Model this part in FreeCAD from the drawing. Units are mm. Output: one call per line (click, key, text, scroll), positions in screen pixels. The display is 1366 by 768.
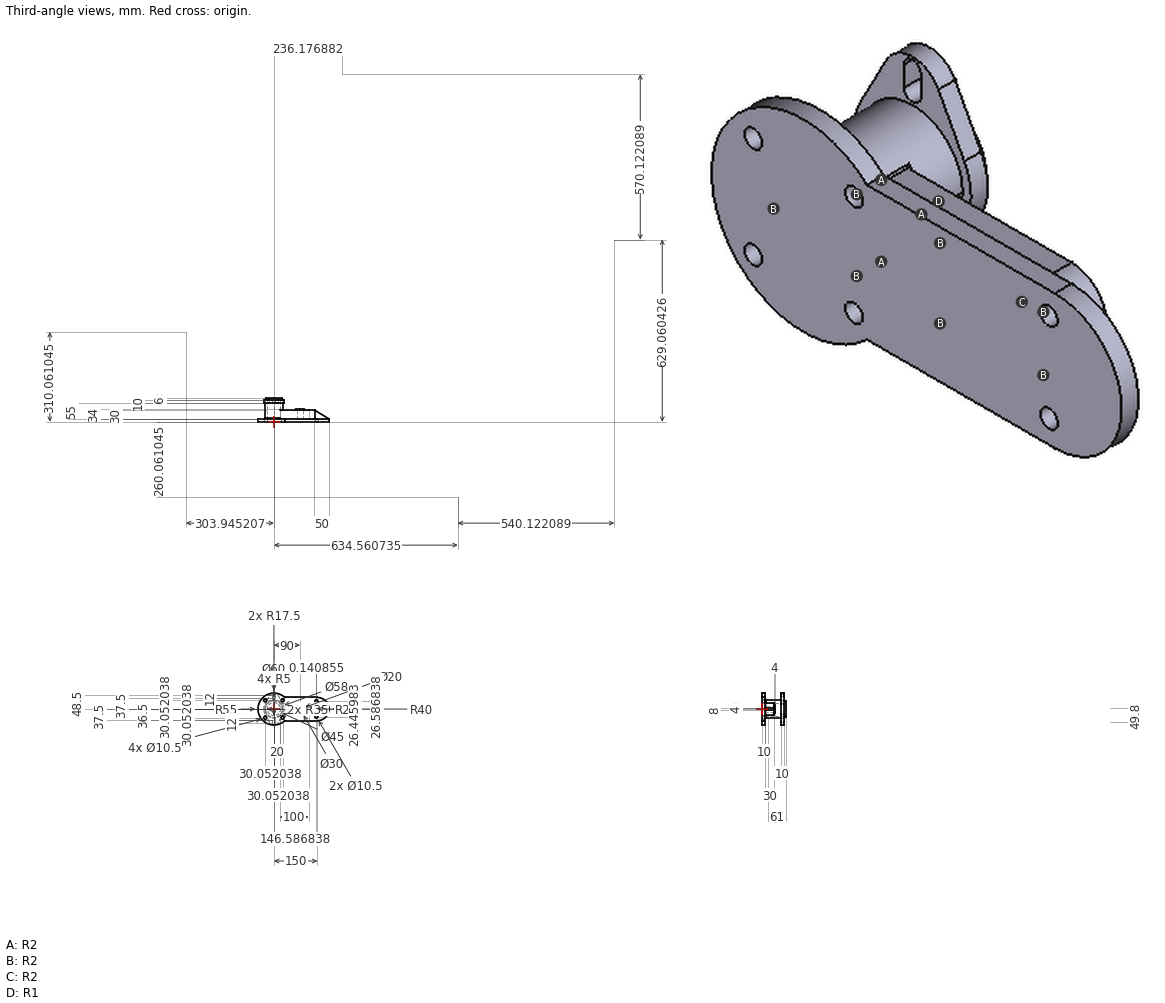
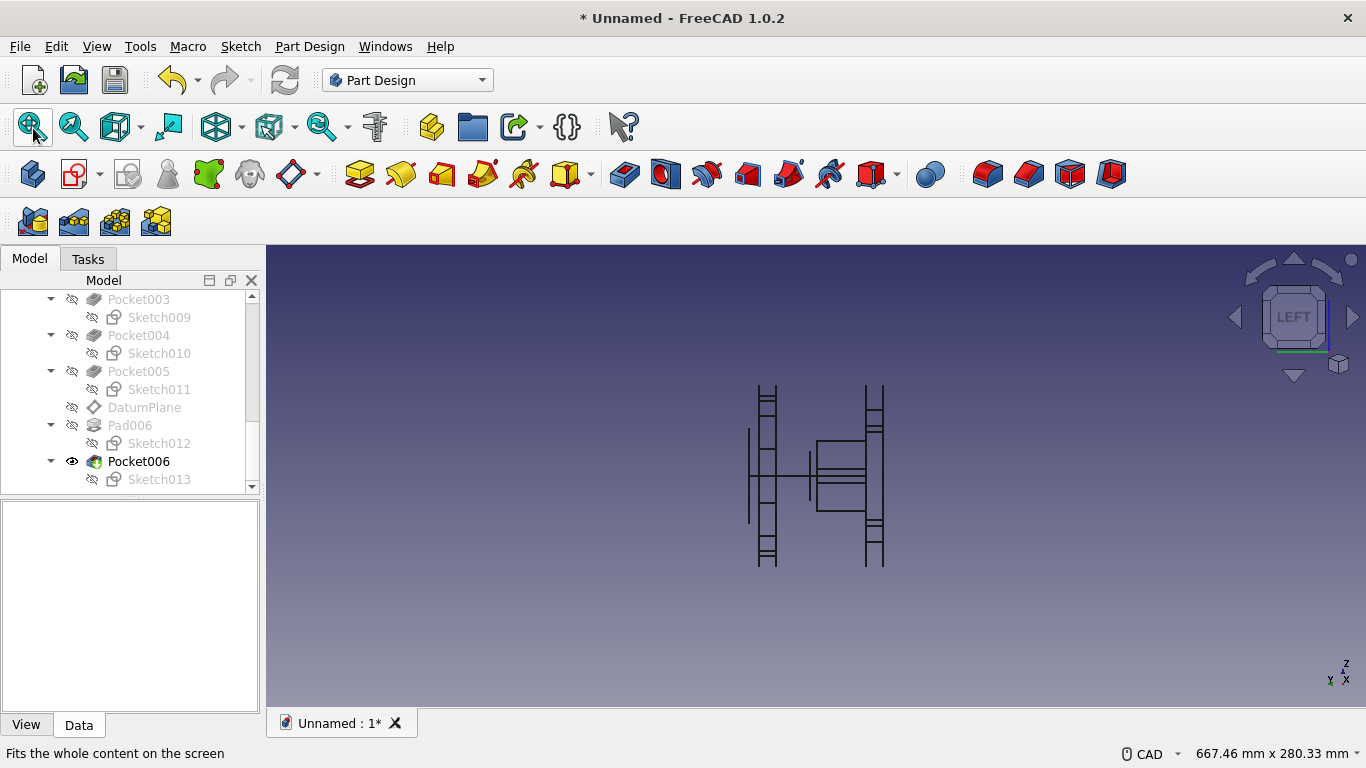
key(0)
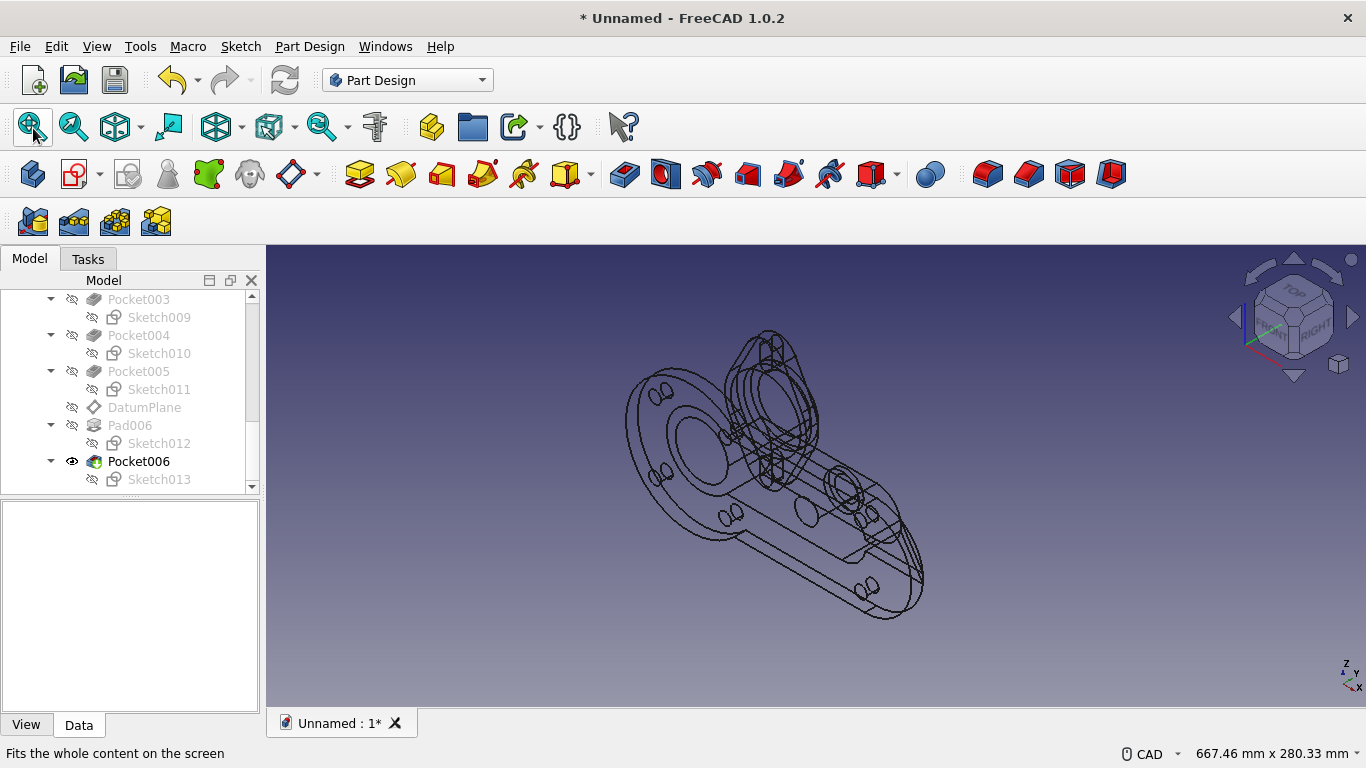
click(757, 418)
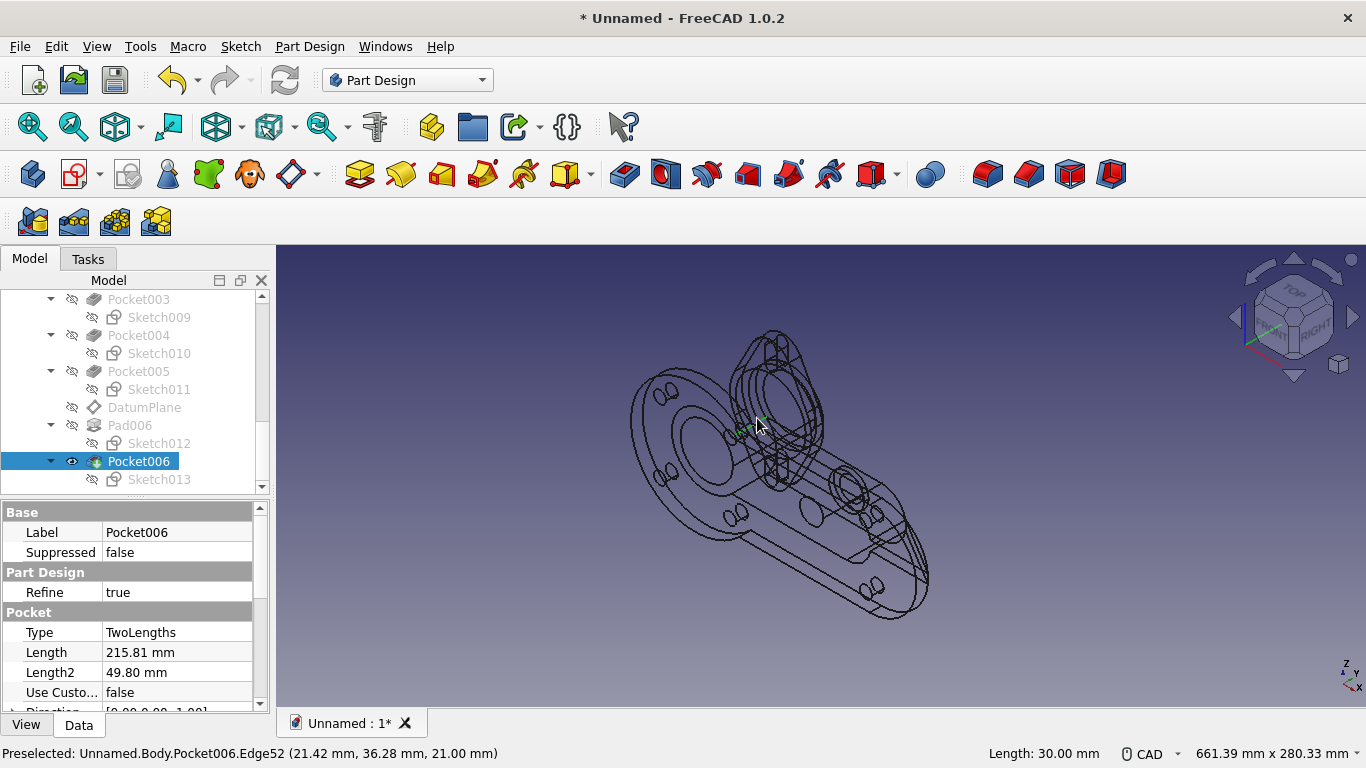
click(749, 483, ctrl)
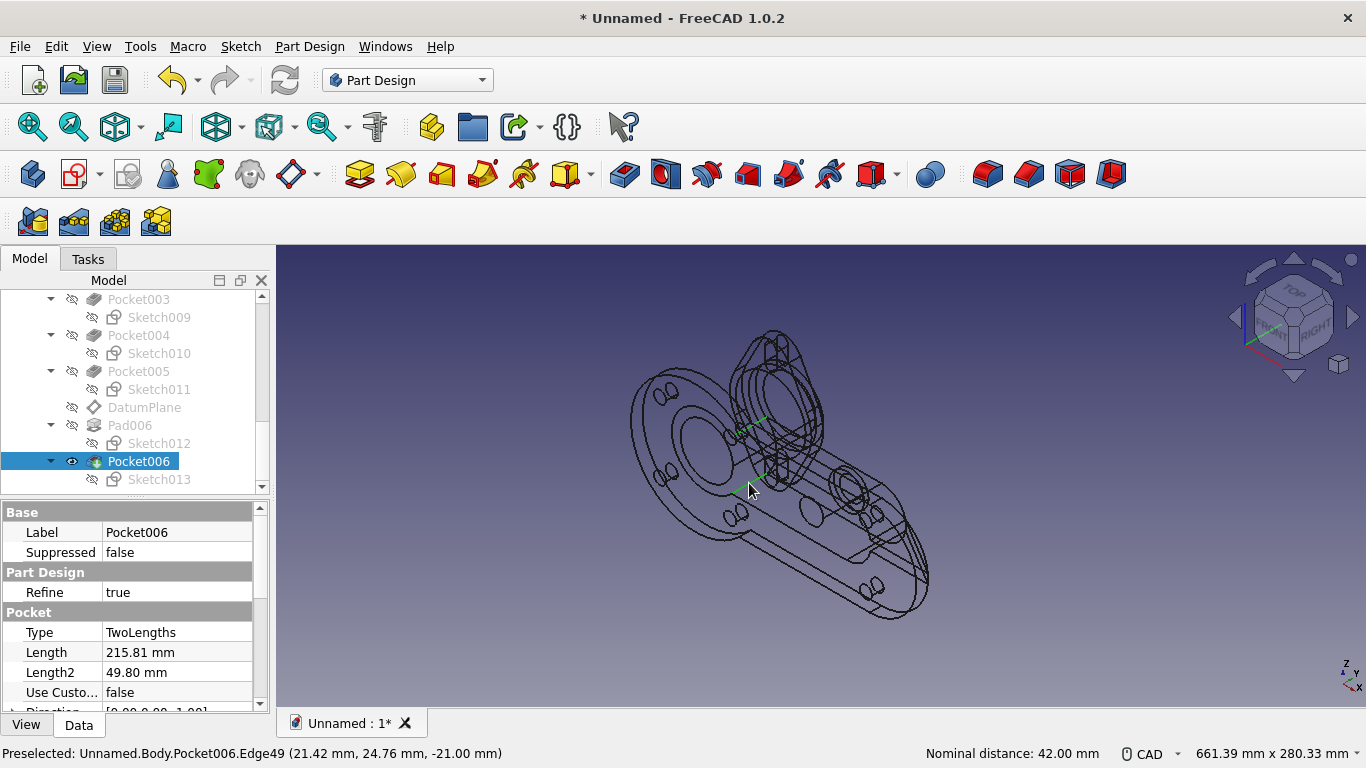
click(772, 468, ctrl)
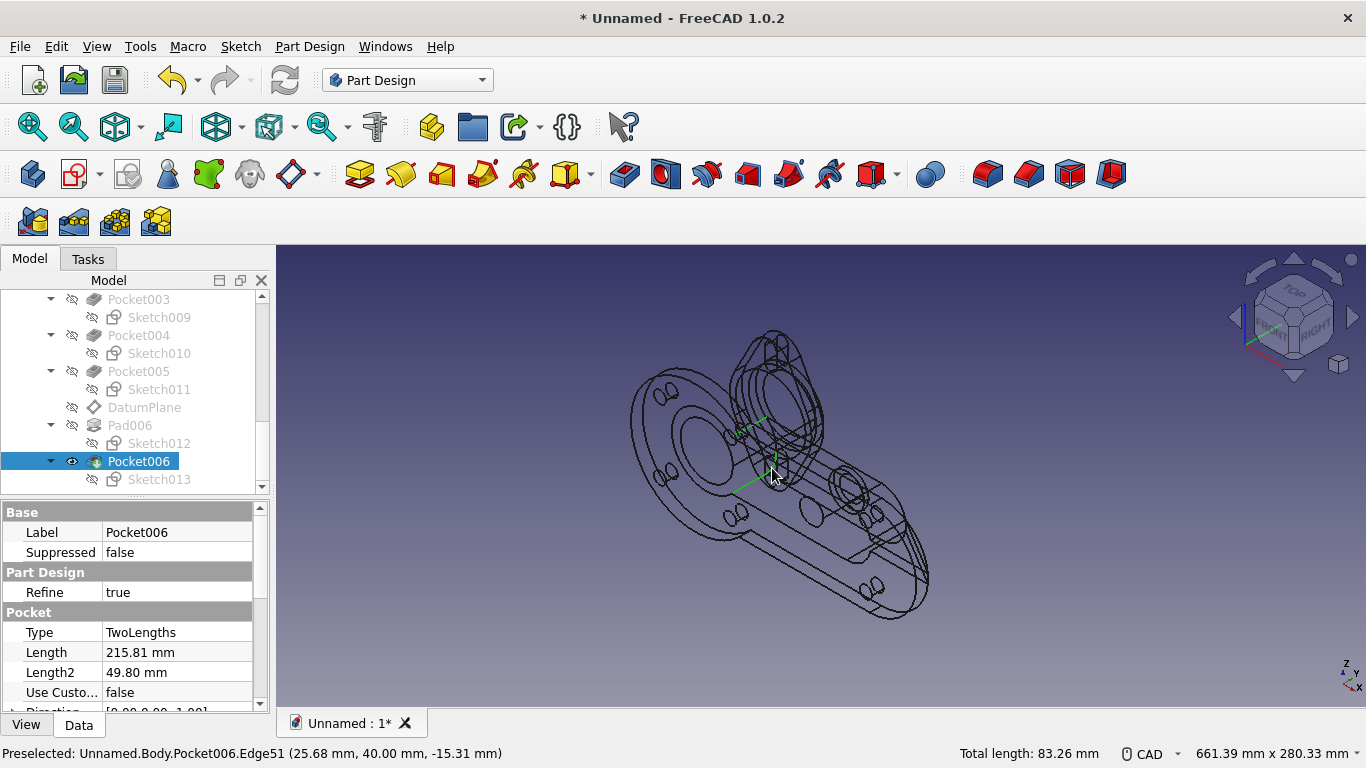
key(v)
key(1)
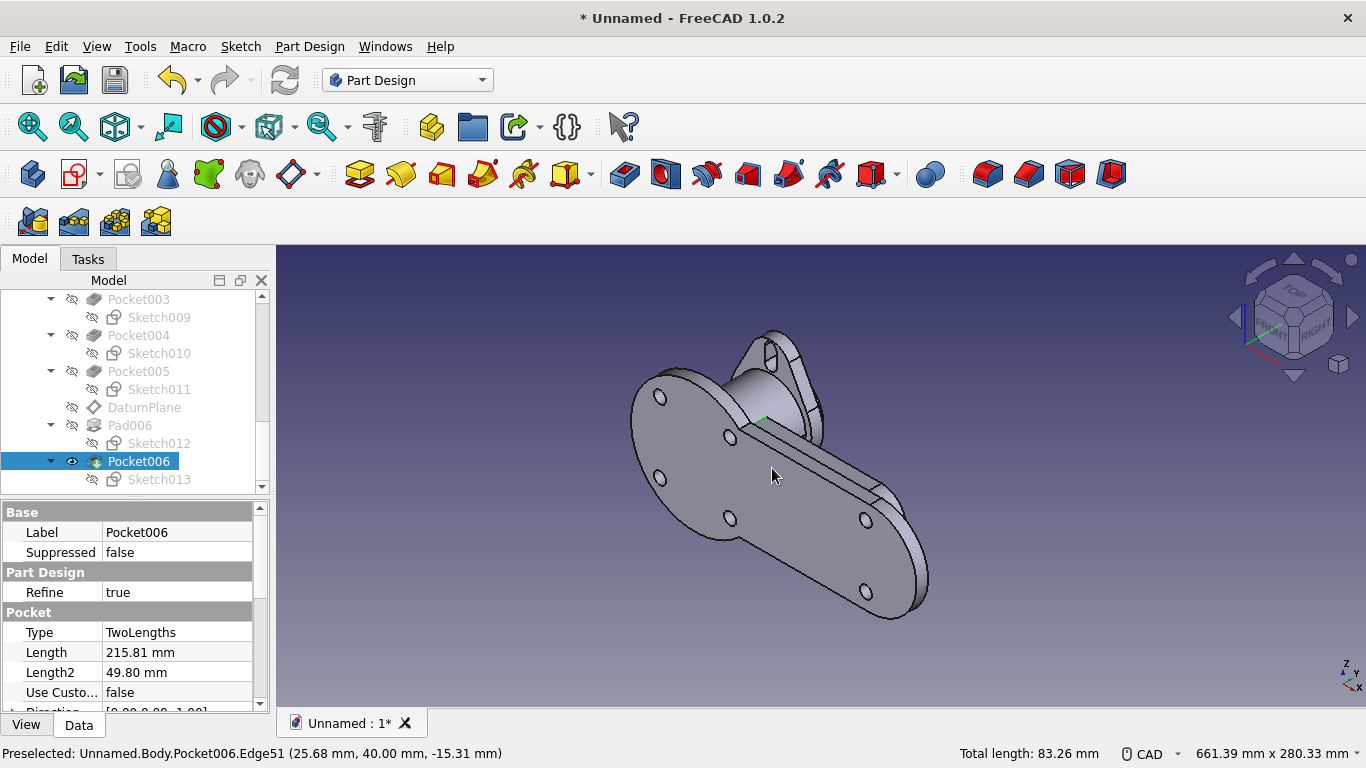
click(988, 174)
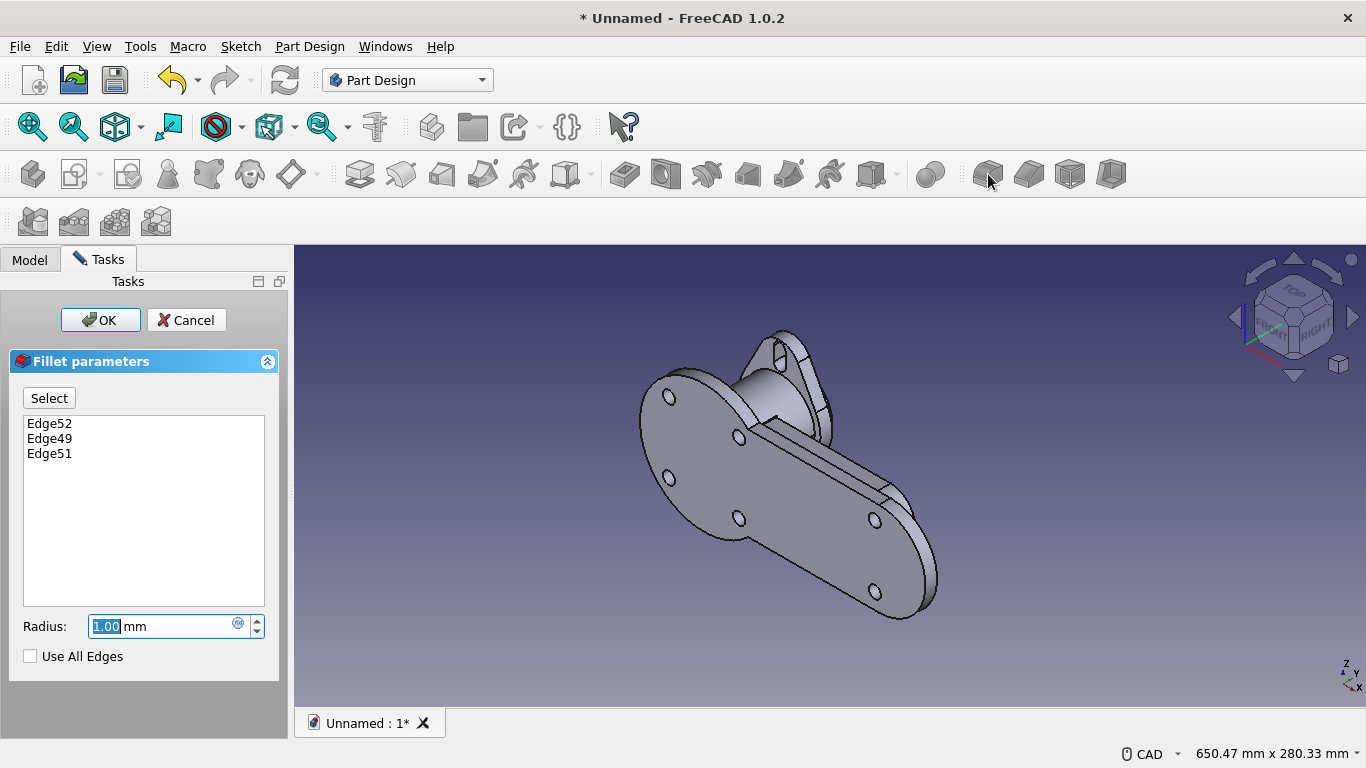
text(2)
key(Tab)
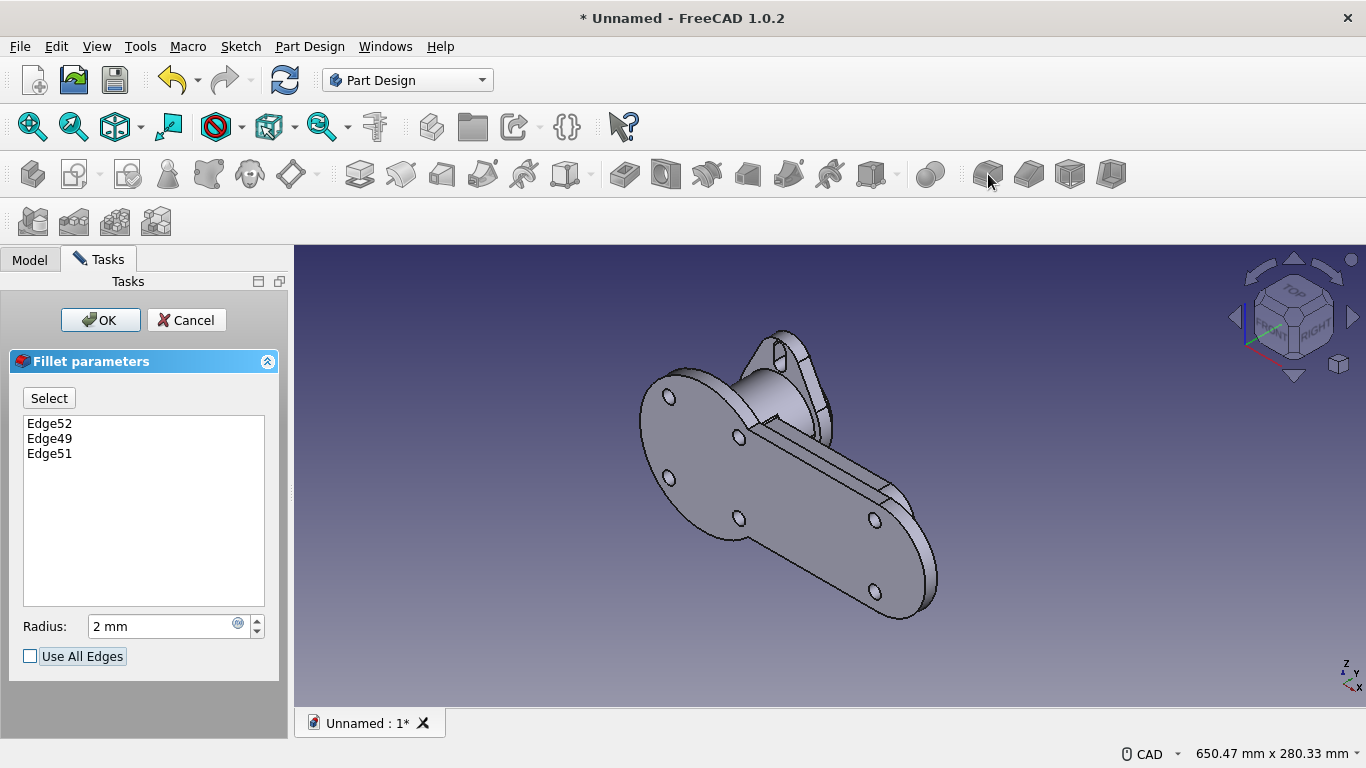
click(101, 320)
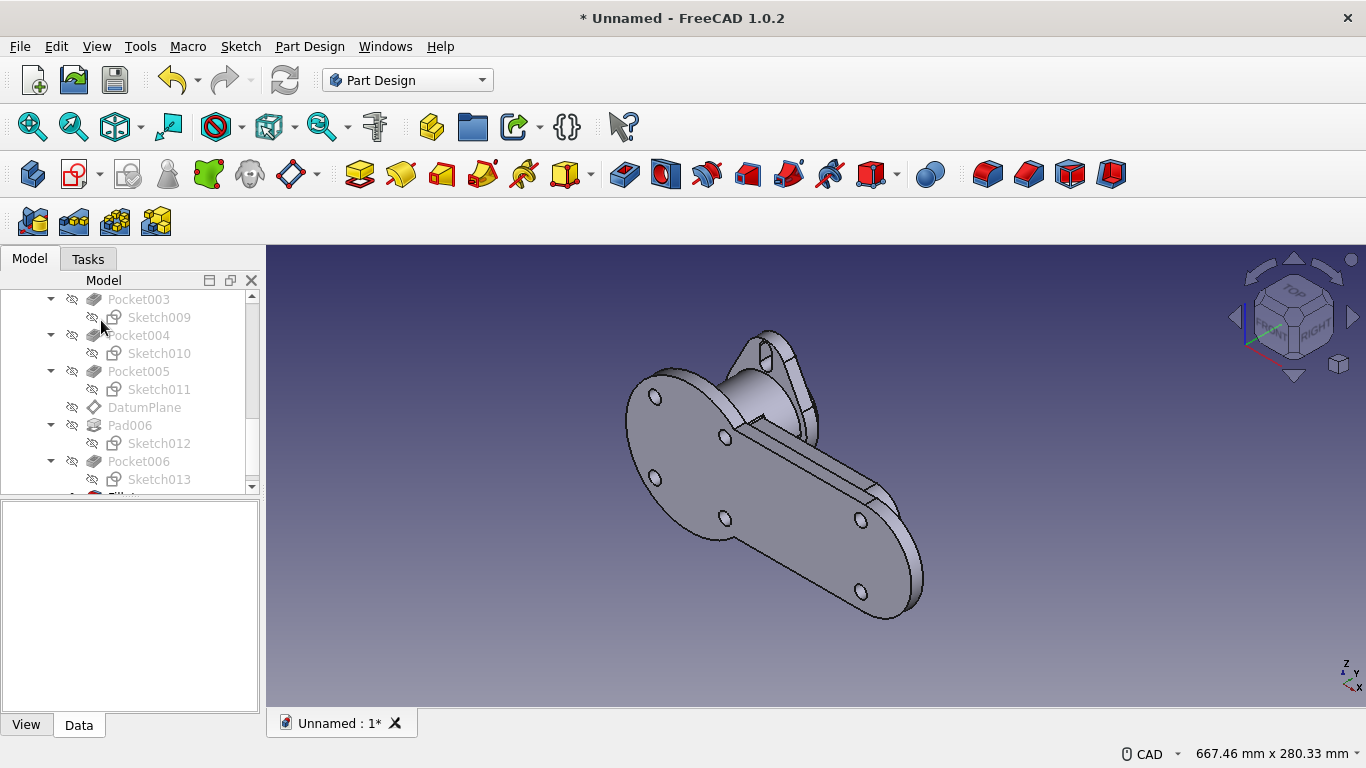
key(2)